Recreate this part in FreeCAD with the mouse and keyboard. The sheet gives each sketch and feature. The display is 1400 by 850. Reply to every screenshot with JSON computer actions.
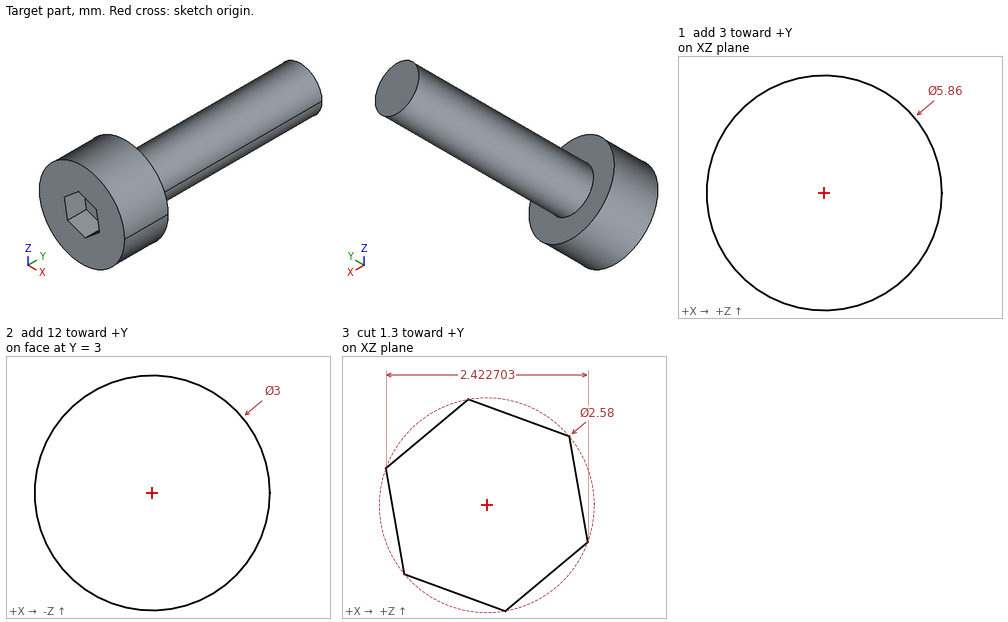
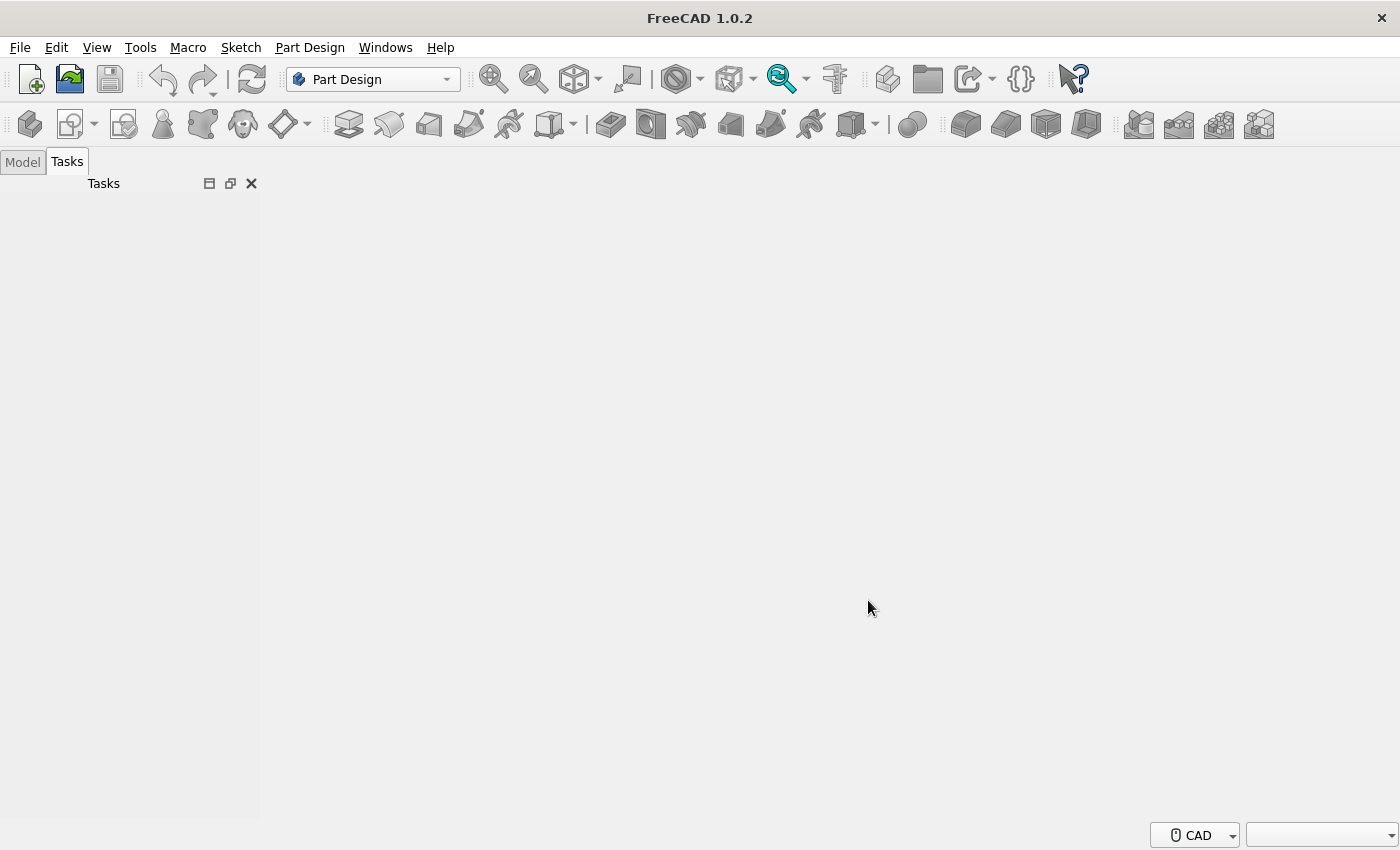
{"action": "left_click", "coordinate": [30, 80]}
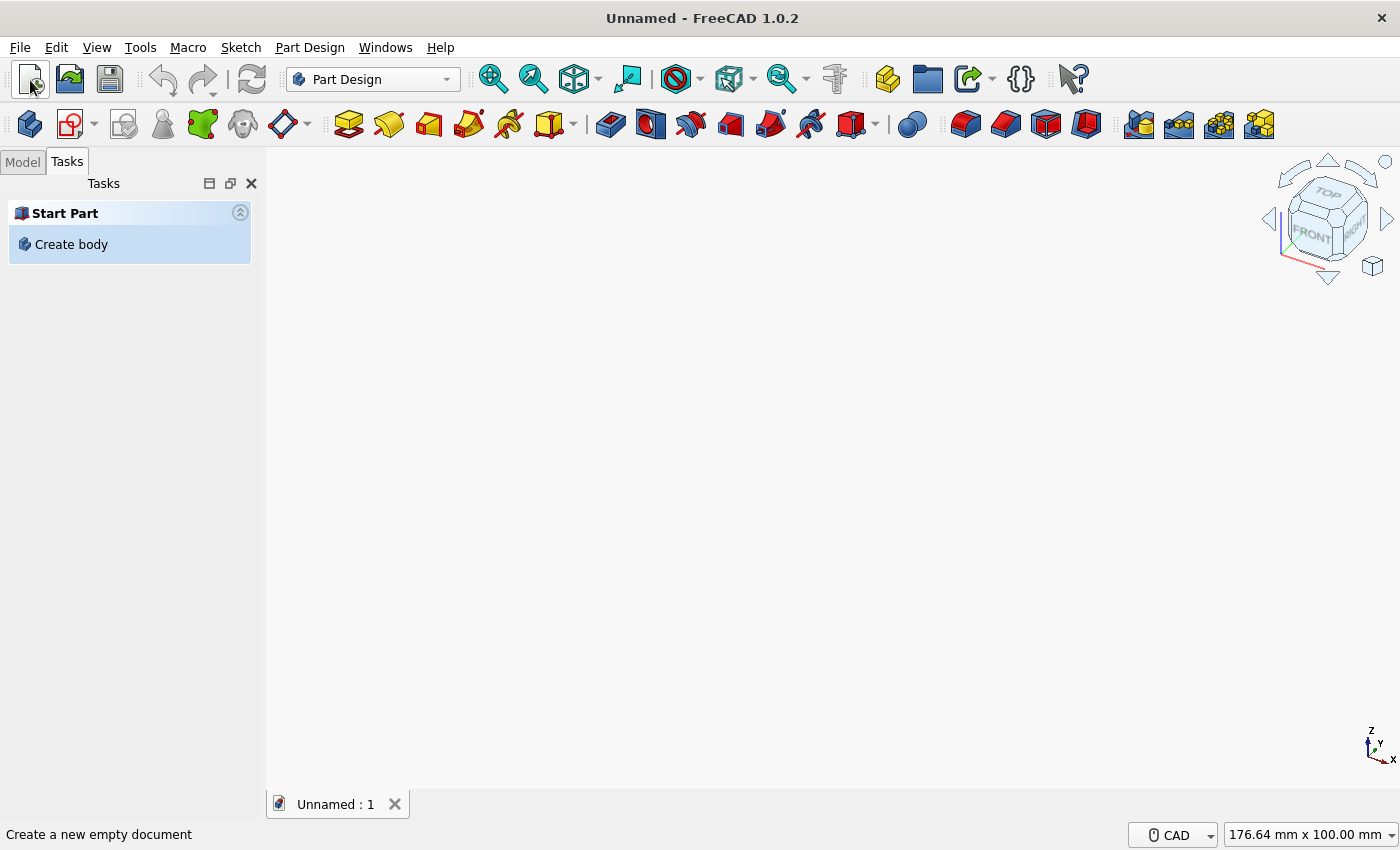
{"action": "left_click", "coordinate": [70, 124]}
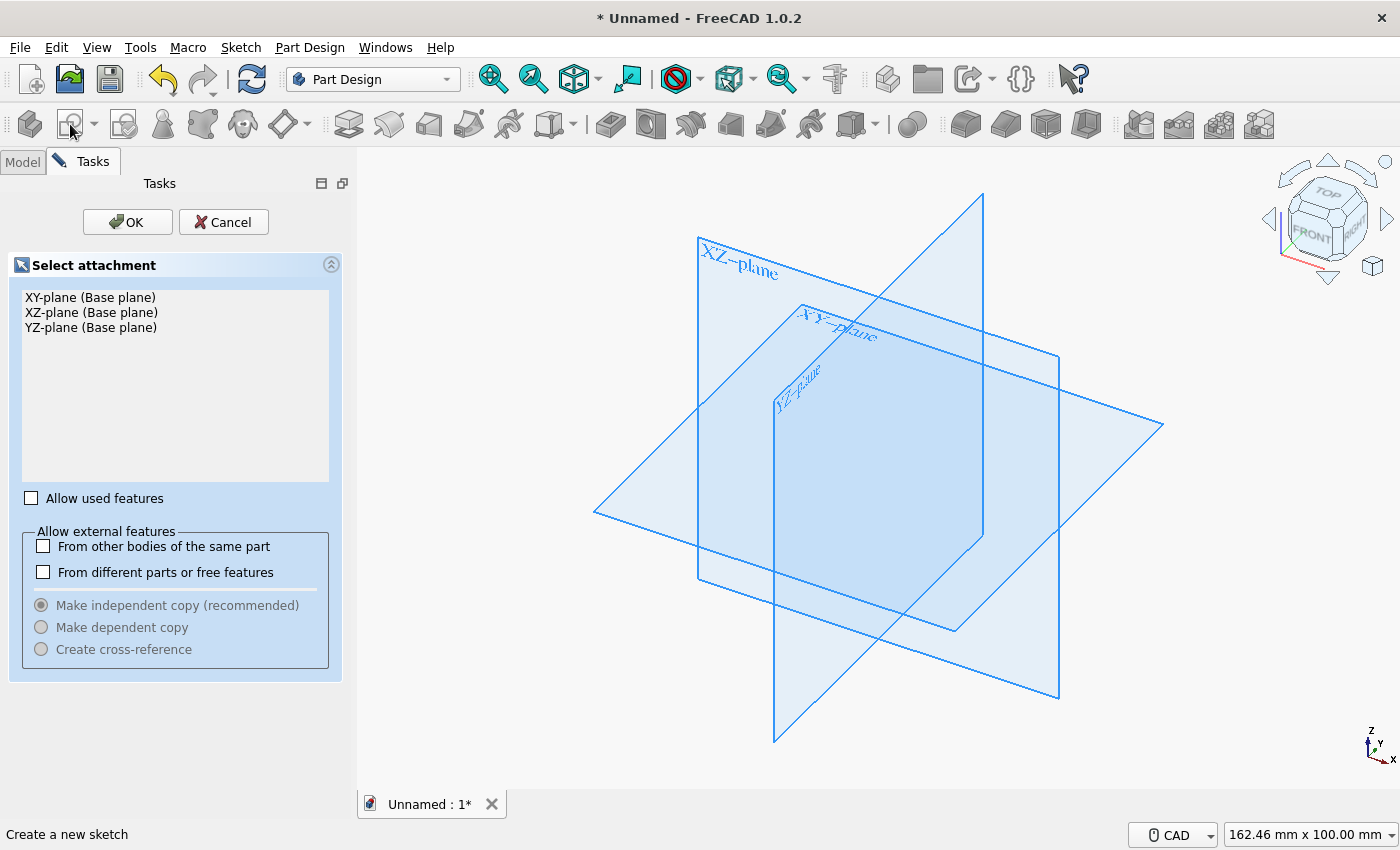
{"action": "left_click", "coordinate": [82, 312]}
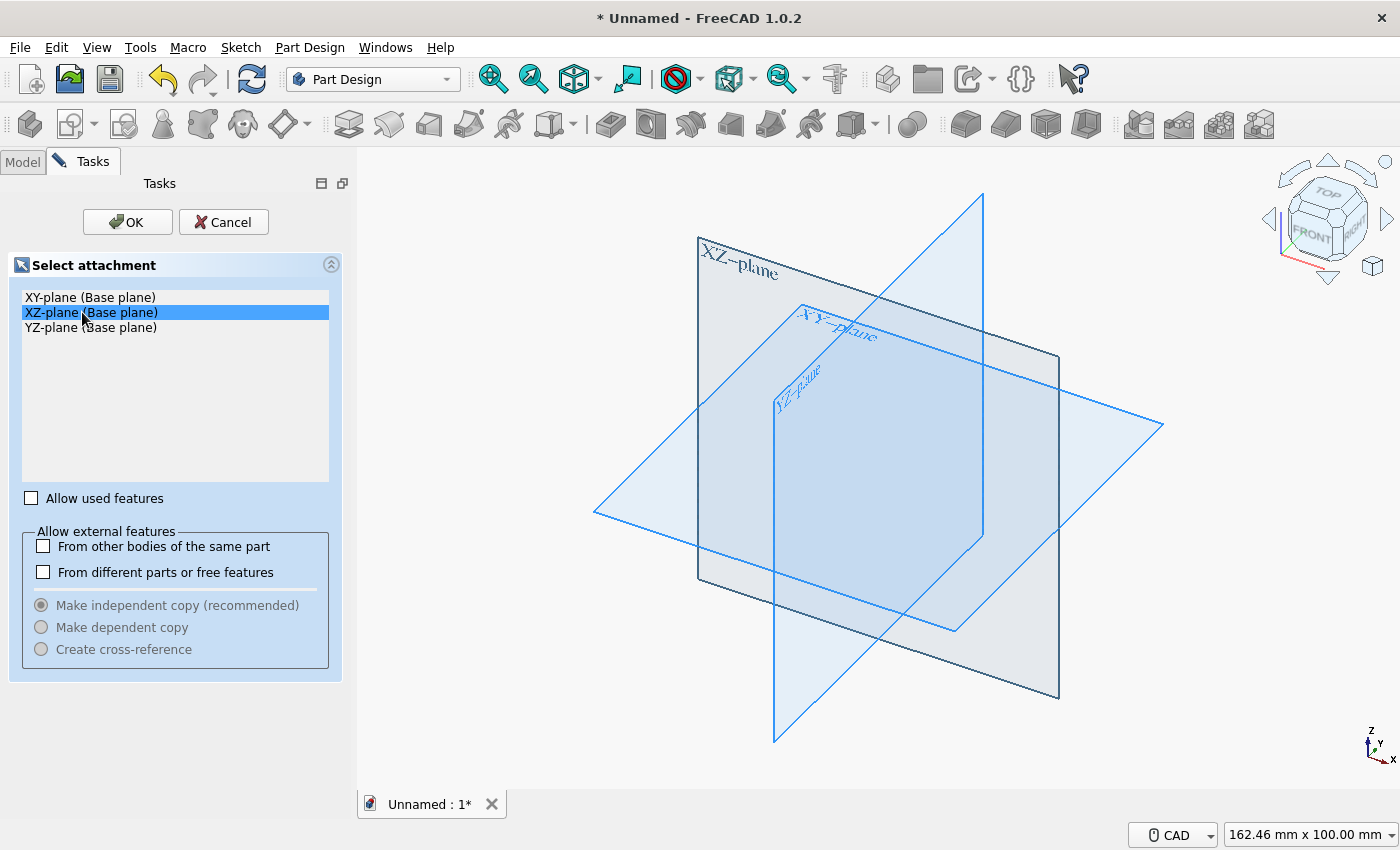
{"action": "left_click", "coordinate": [128, 222]}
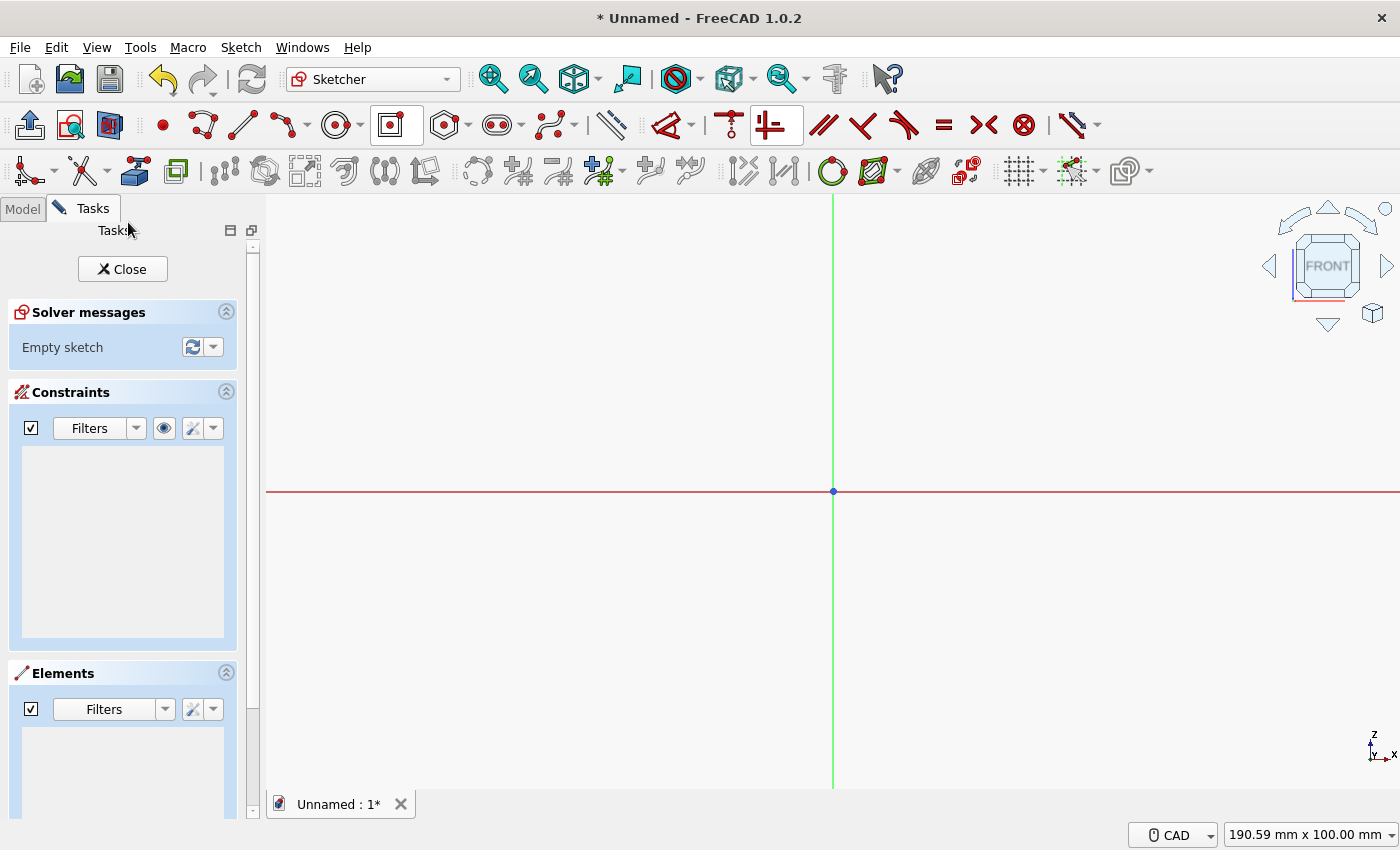
{"action": "scroll", "coordinate": [840, 492], "scroll_direction": "up", "scroll_amount": 12}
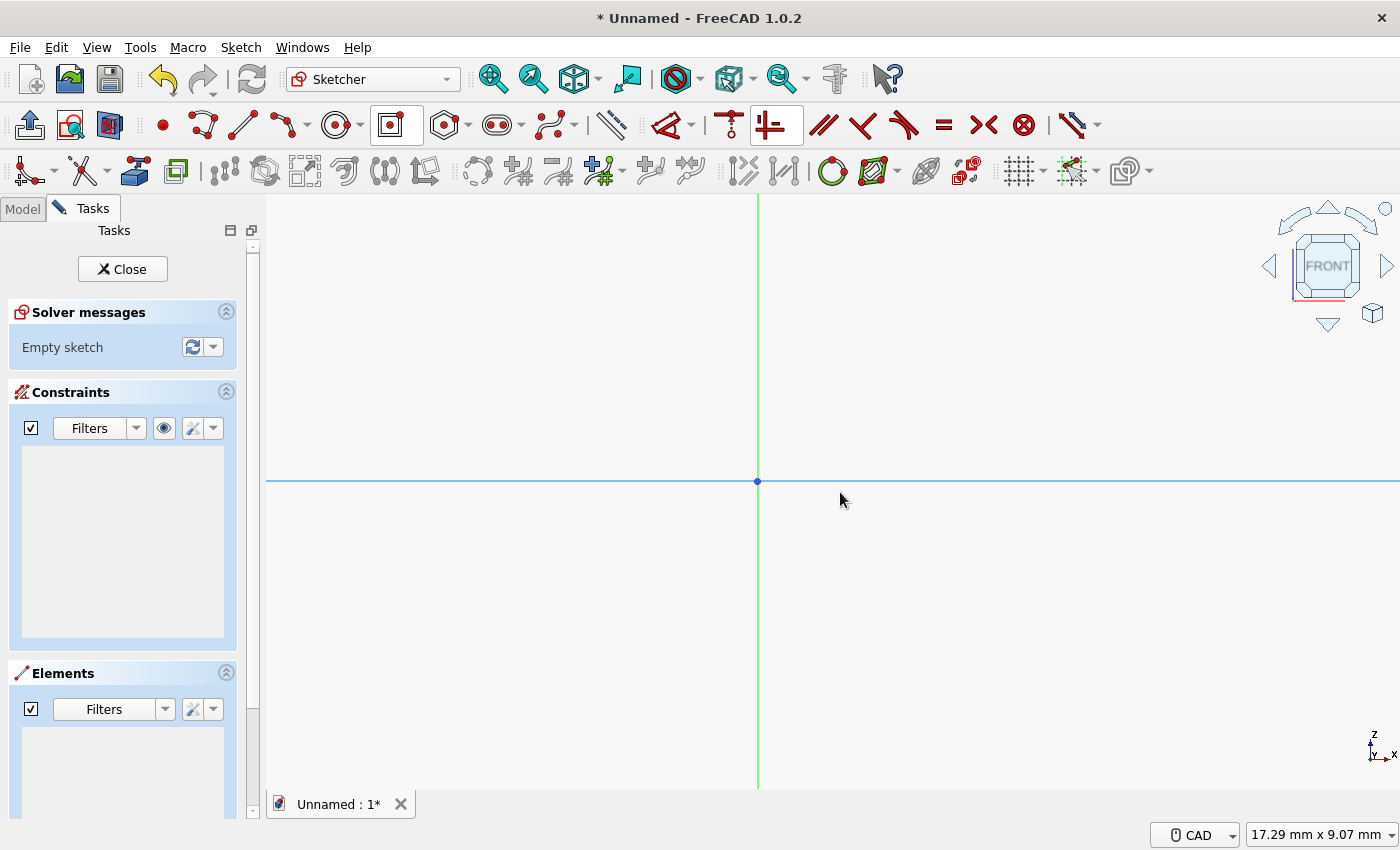
{"action": "left_click", "coordinate": [336, 126]}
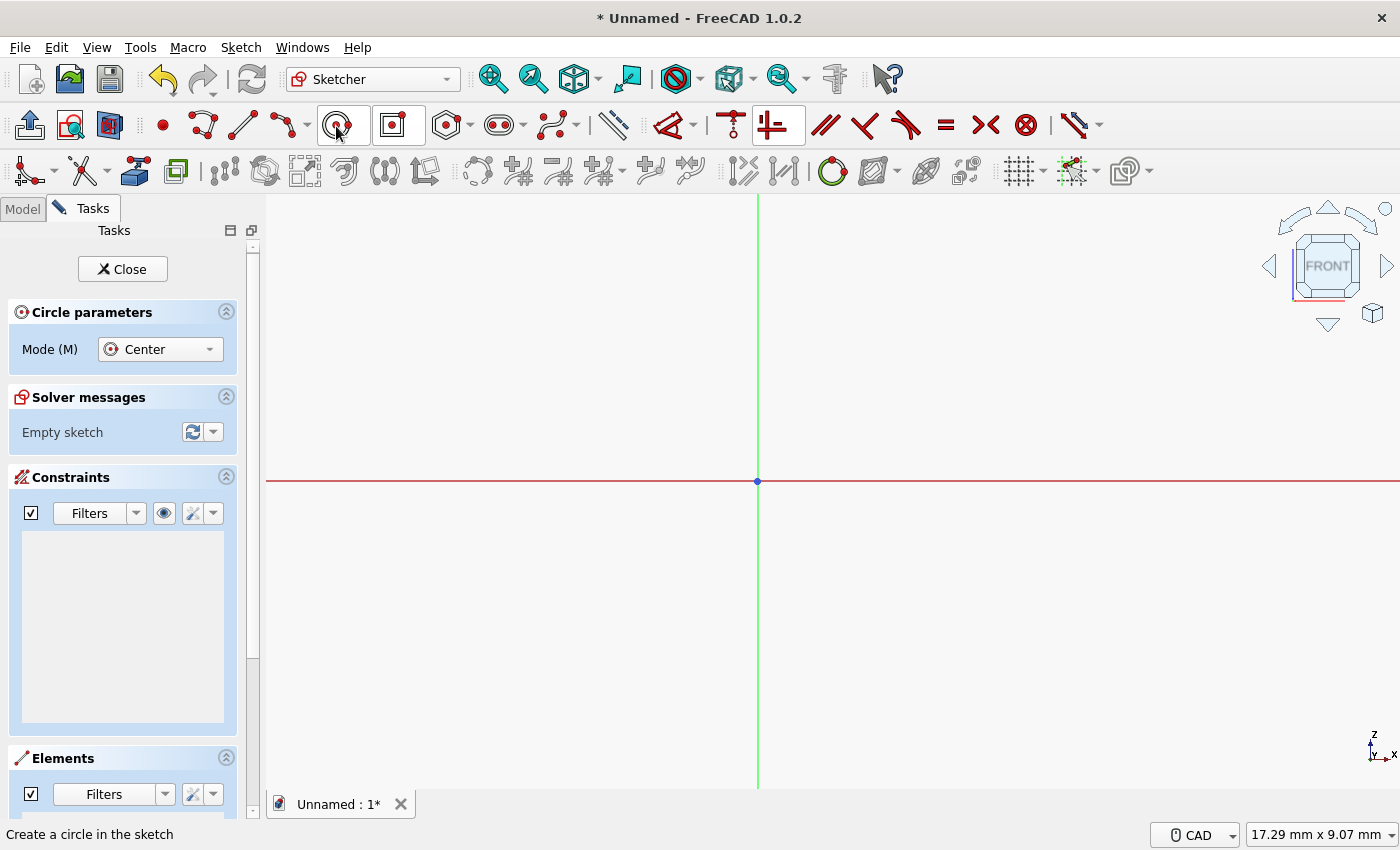
{"action": "left_click", "coordinate": [758, 481]}
{"action": "mouse_move", "coordinate": [894, 346]}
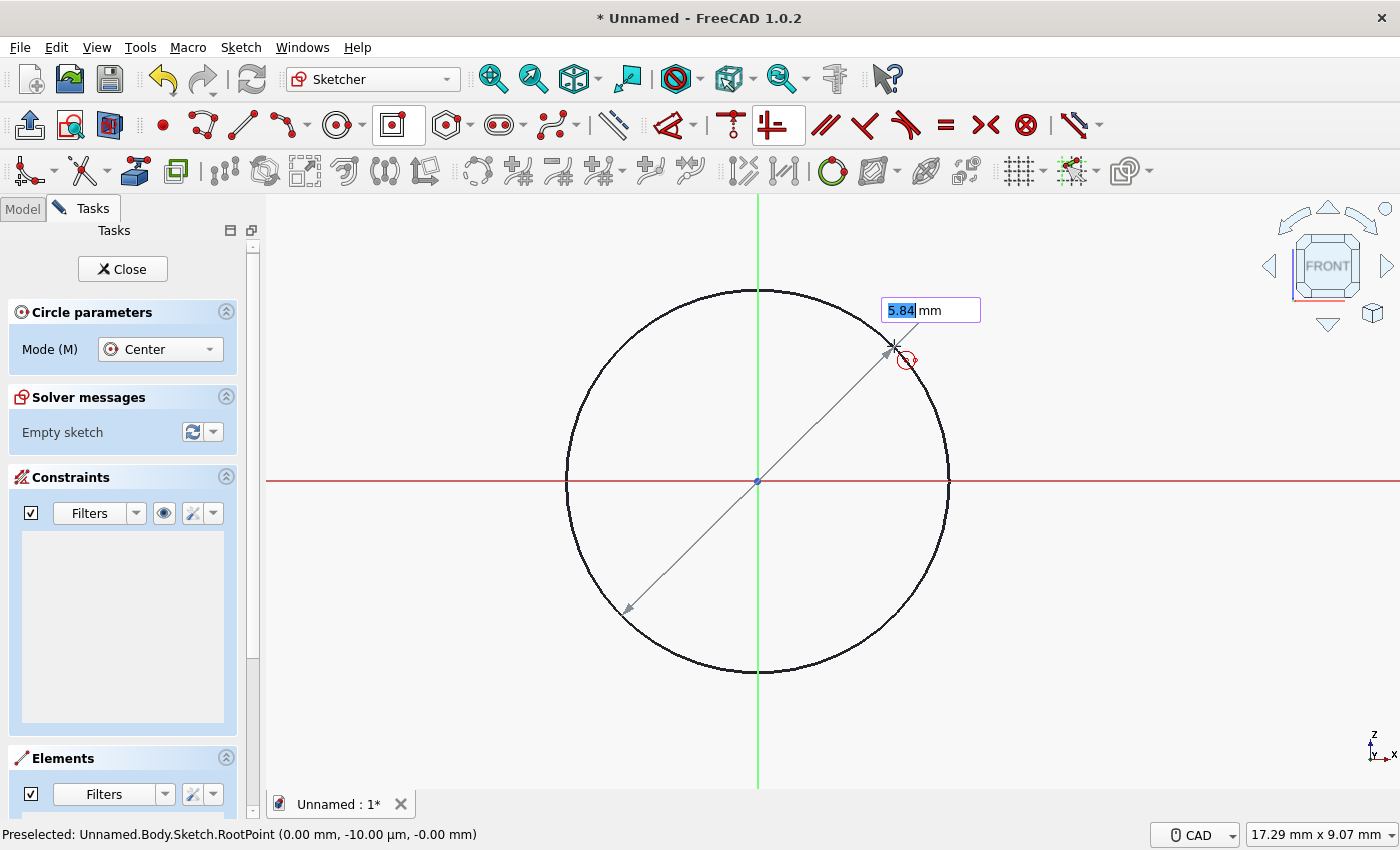
{"action": "type", "text": "5.86"}
{"action": "key", "text": "Return"}
{"action": "key", "text": "Escape"}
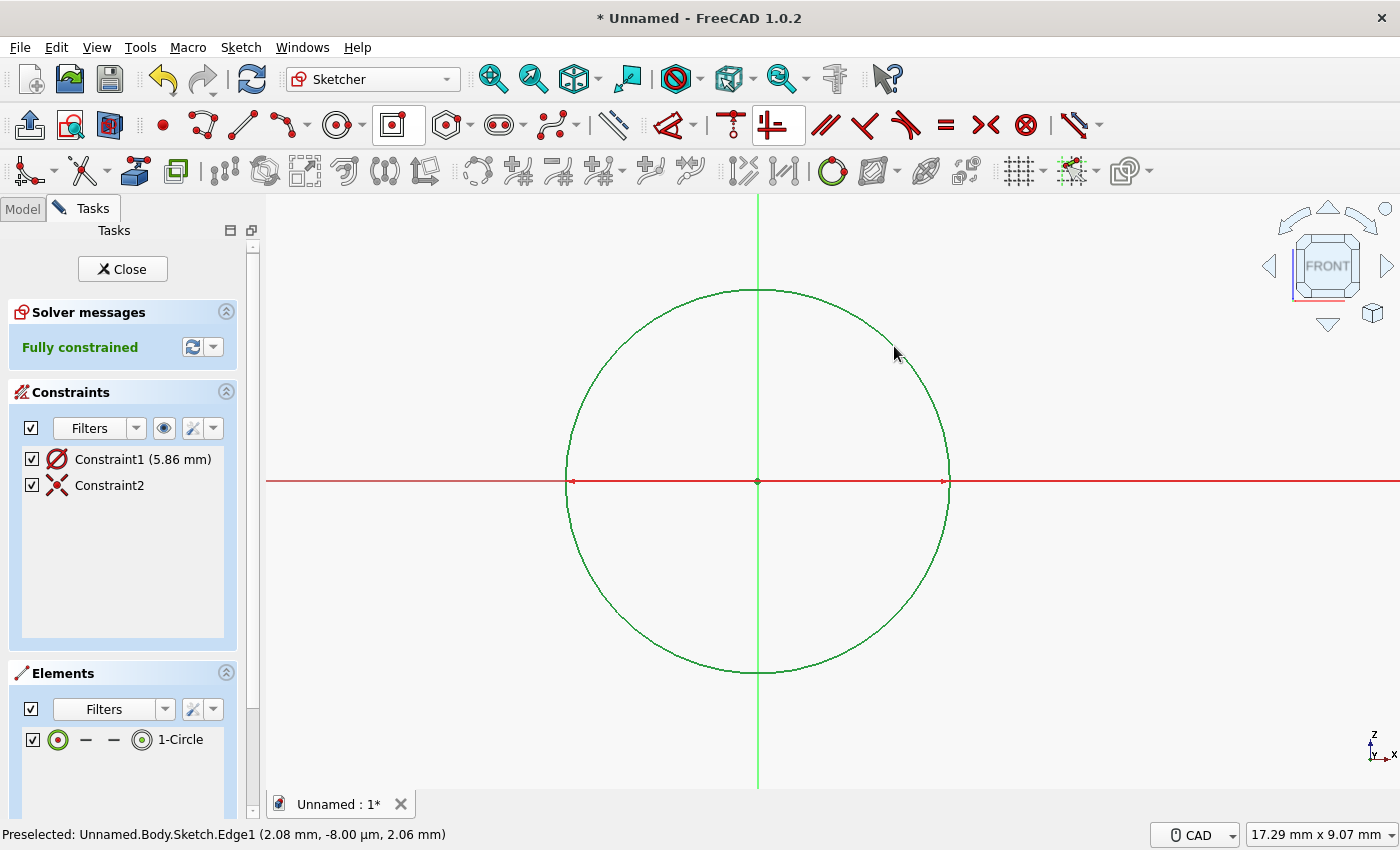
{"action": "left_click", "coordinate": [123, 269]}